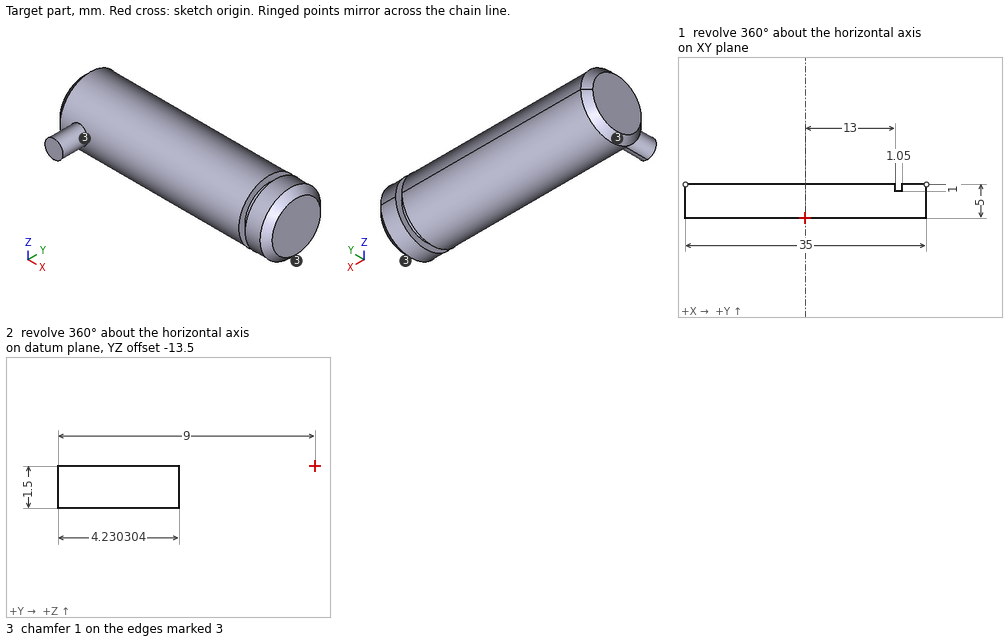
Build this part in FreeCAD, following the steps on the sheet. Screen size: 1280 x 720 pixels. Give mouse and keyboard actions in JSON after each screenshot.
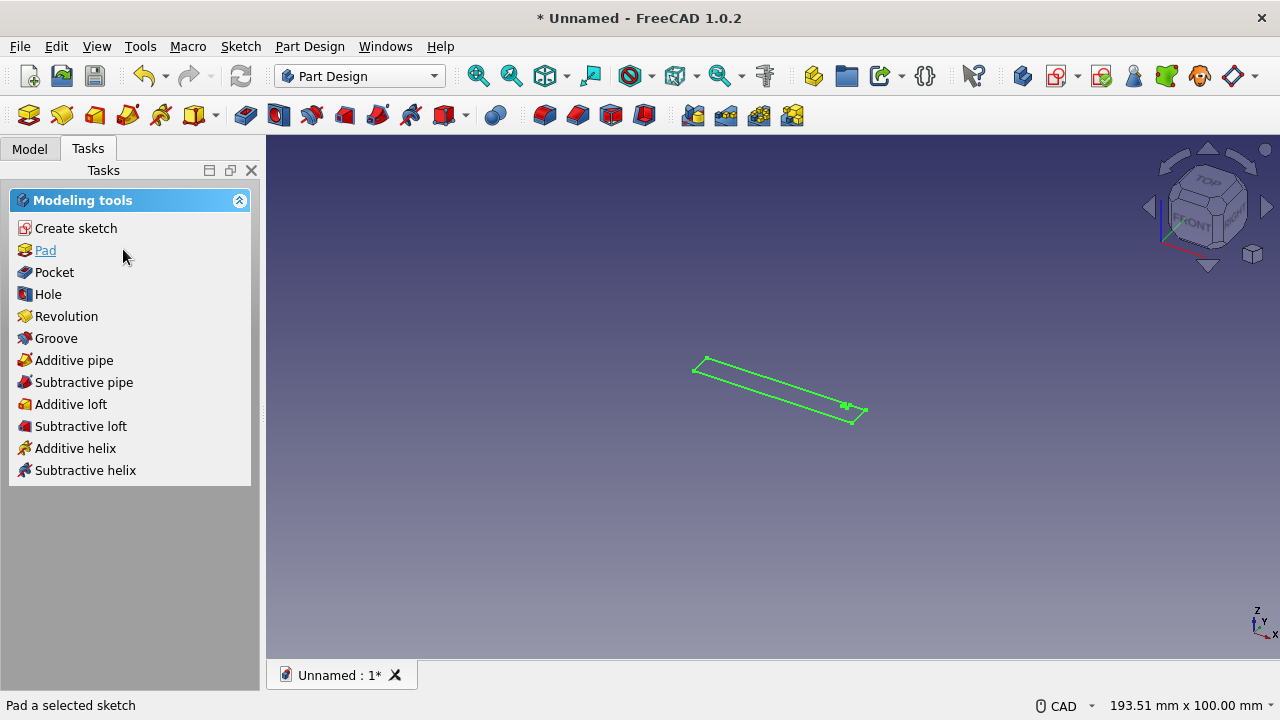
{"action": "left_click", "coordinate": [62, 116]}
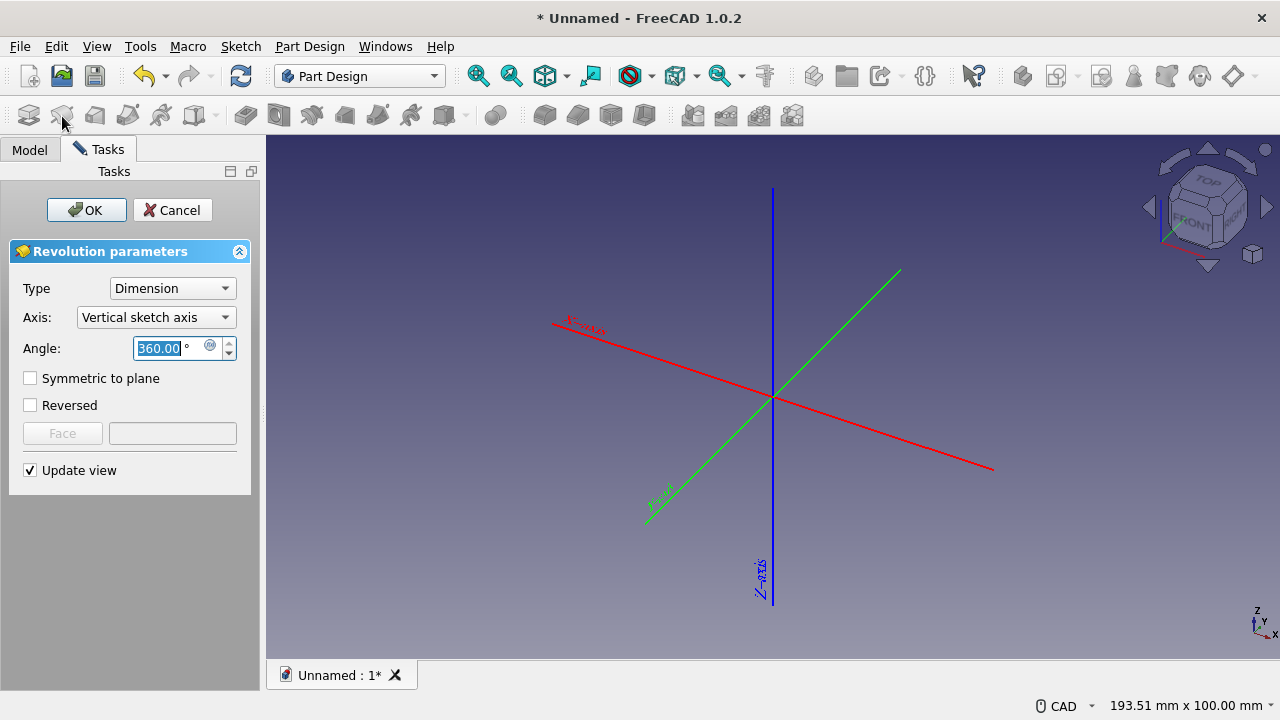
{"action": "left_click", "coordinate": [157, 318]}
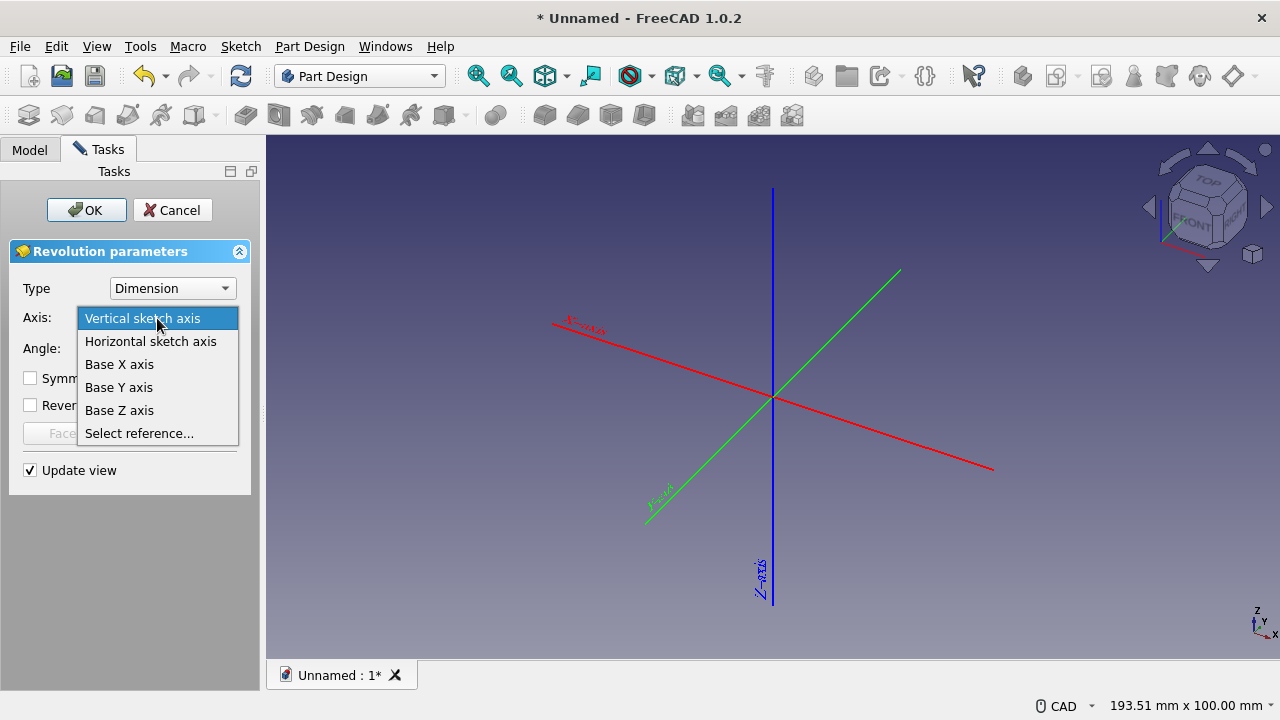
{"action": "left_click", "coordinate": [156, 342]}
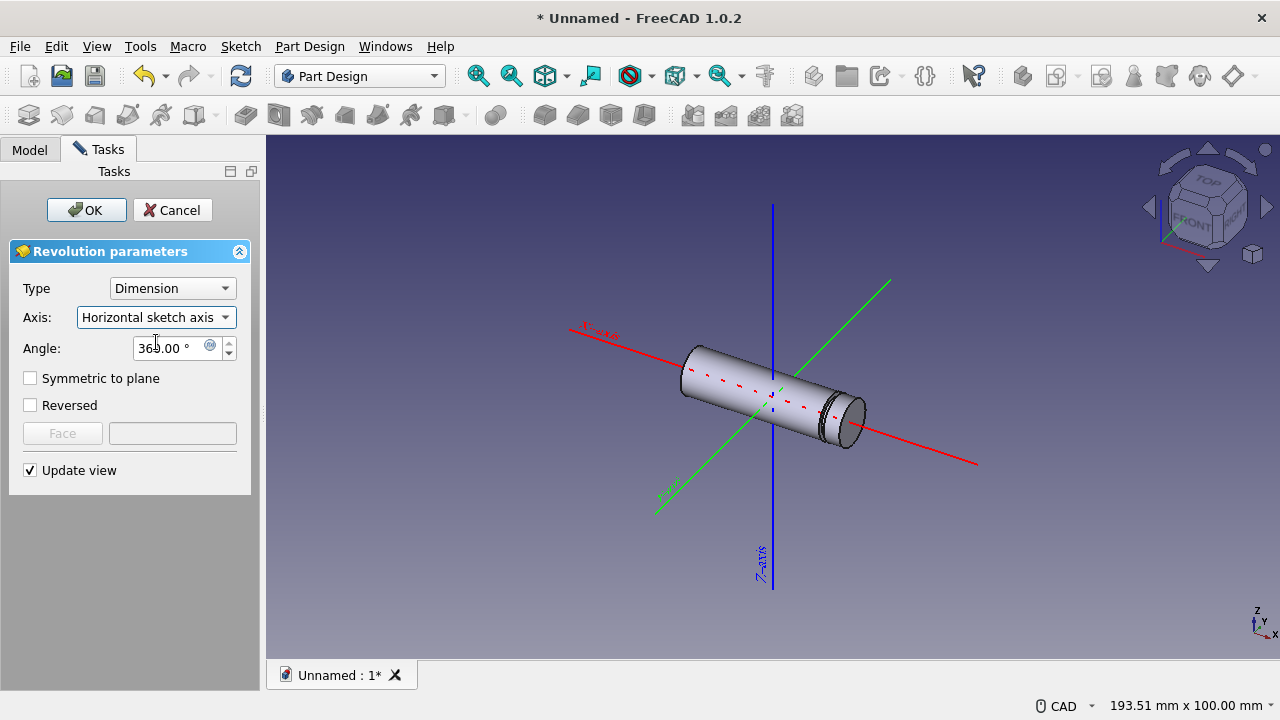
{"action": "left_click", "coordinate": [87, 210]}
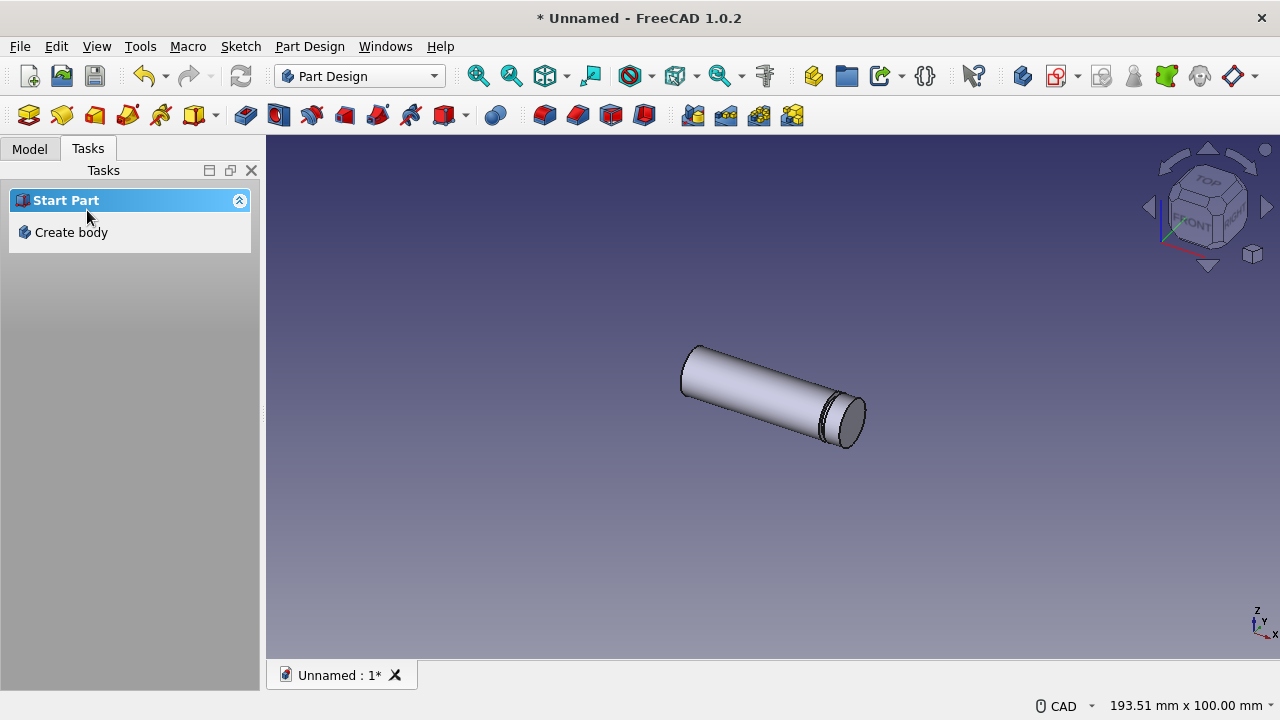
{"action": "left_click", "coordinate": [479, 76]}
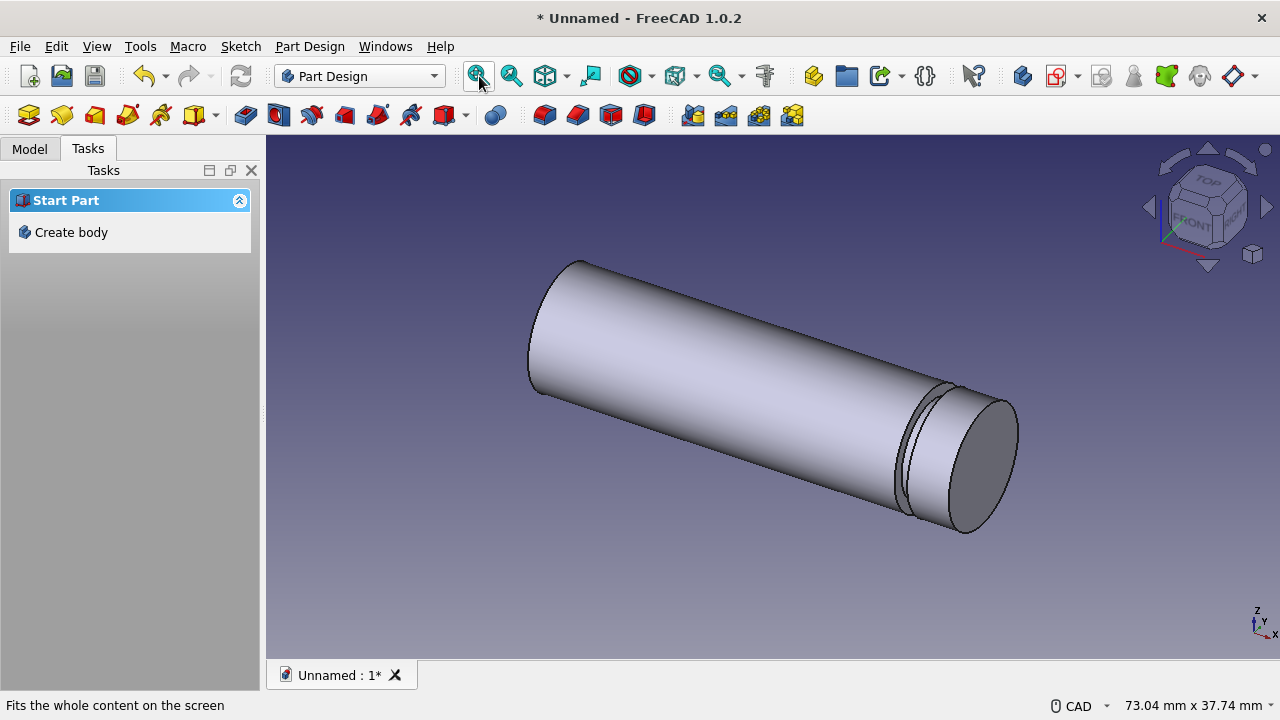
{"action": "left_click", "coordinate": [30, 148]}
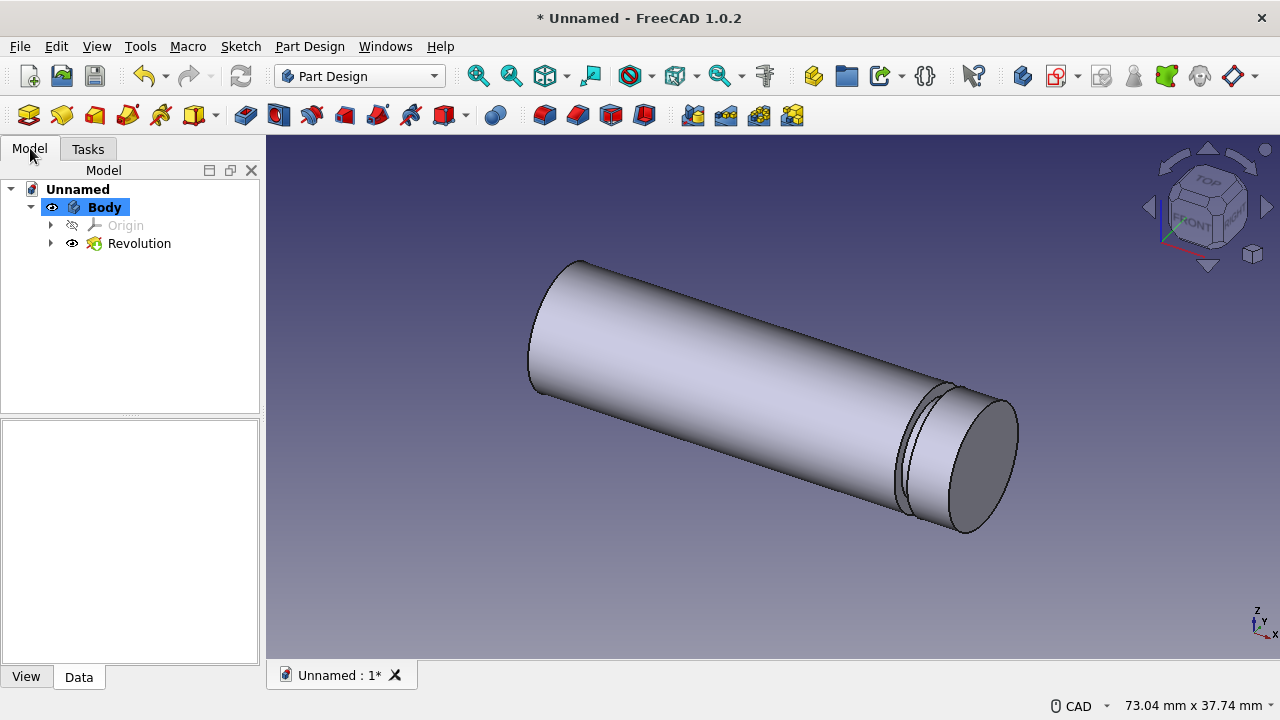
{"action": "left_click", "coordinate": [51, 225]}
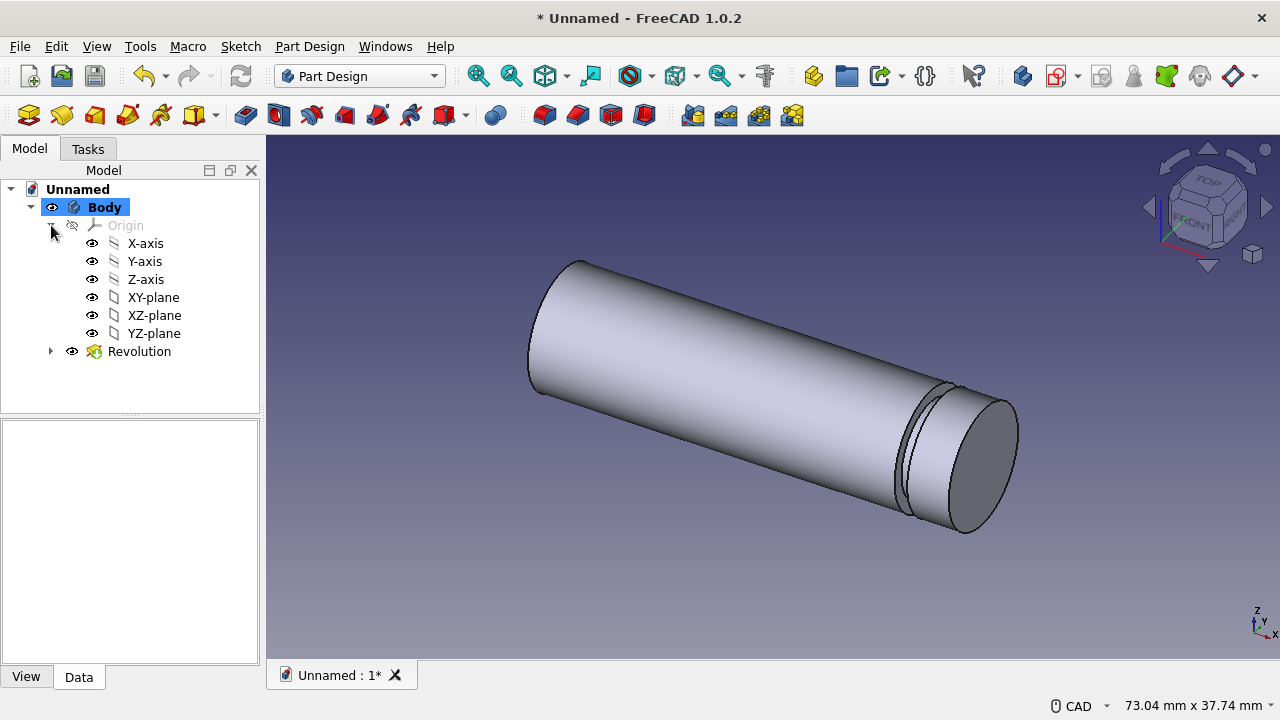
{"action": "left_click", "coordinate": [137, 333]}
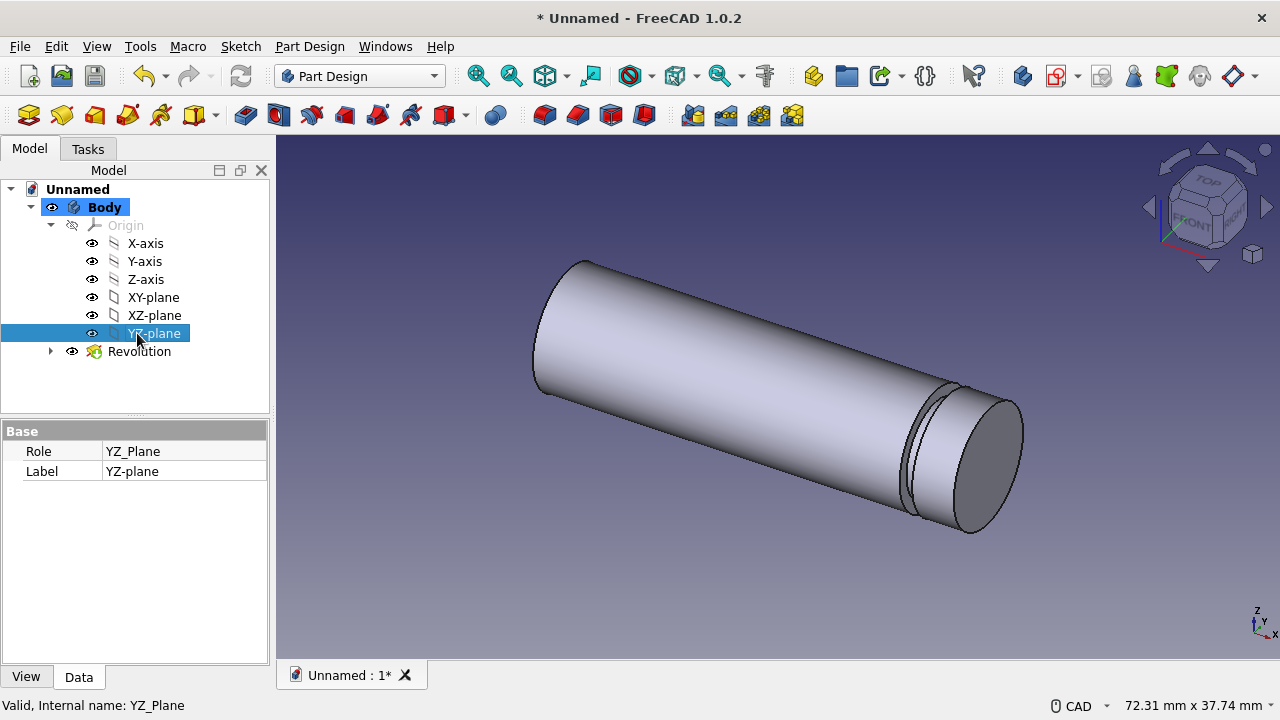
{"action": "left_click", "coordinate": [1232, 76]}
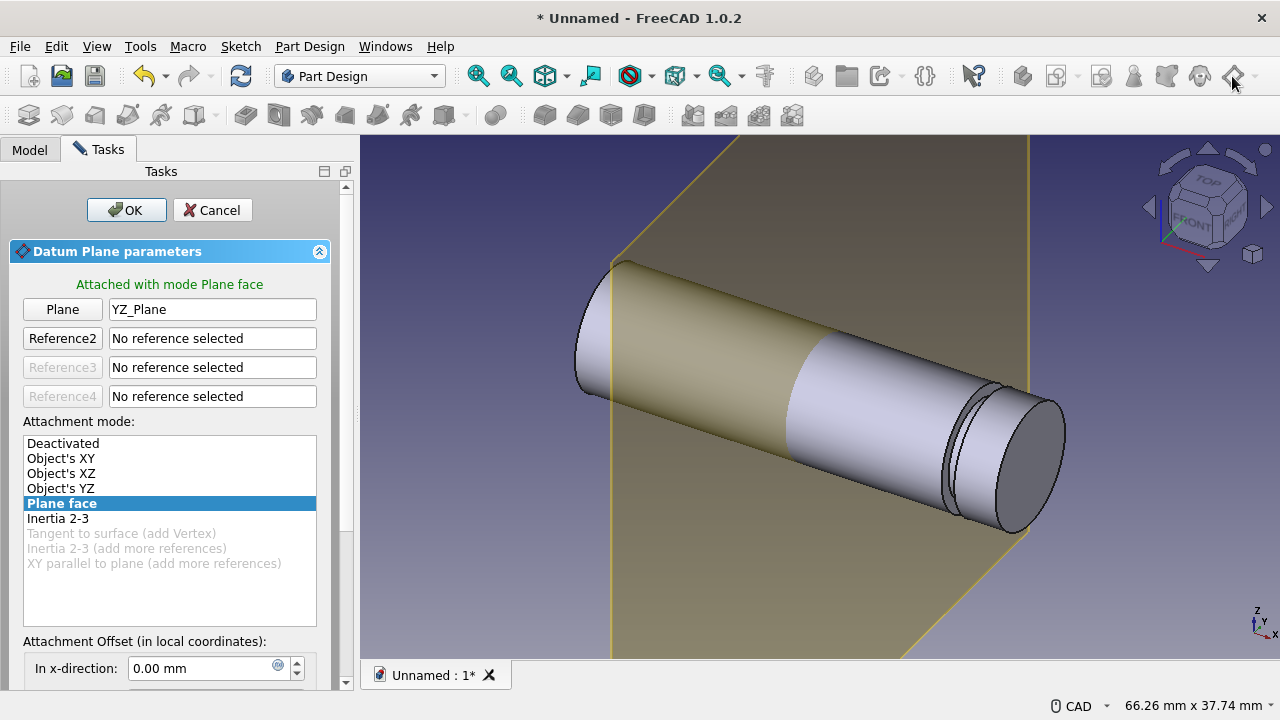
{"action": "scroll", "coordinate": [346, 436], "scroll_direction": "down", "scroll_amount": 2}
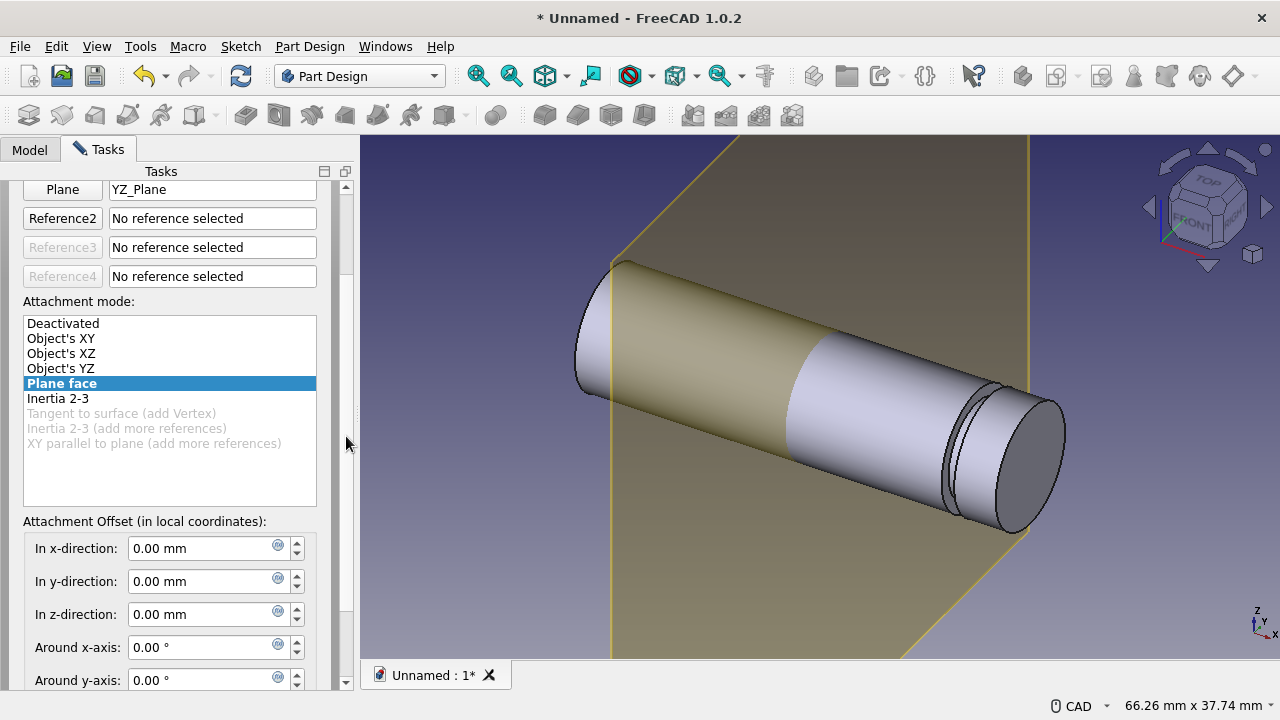
{"action": "triple_click", "coordinate": [210, 614]}